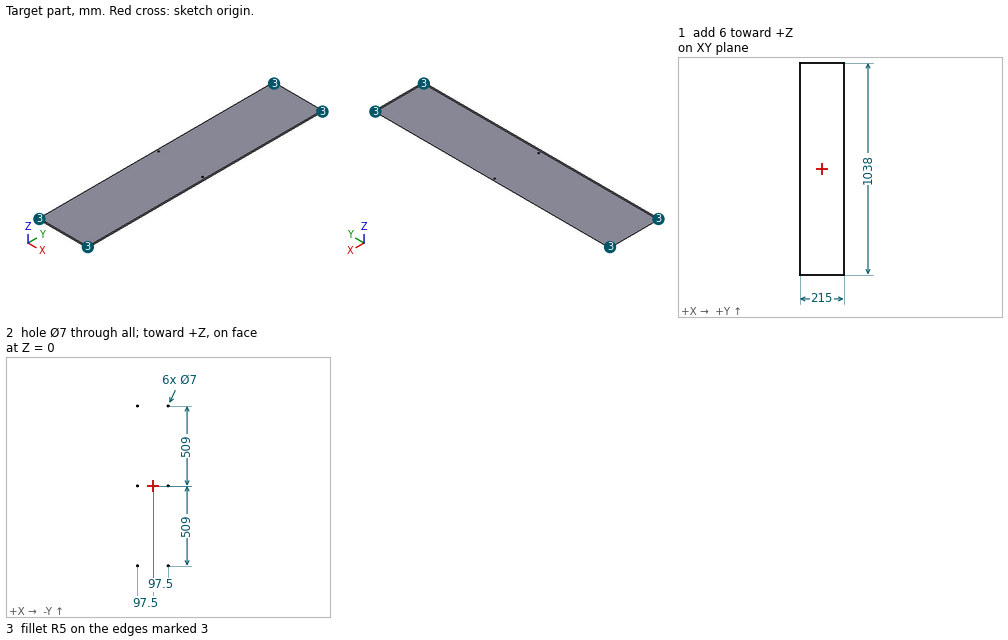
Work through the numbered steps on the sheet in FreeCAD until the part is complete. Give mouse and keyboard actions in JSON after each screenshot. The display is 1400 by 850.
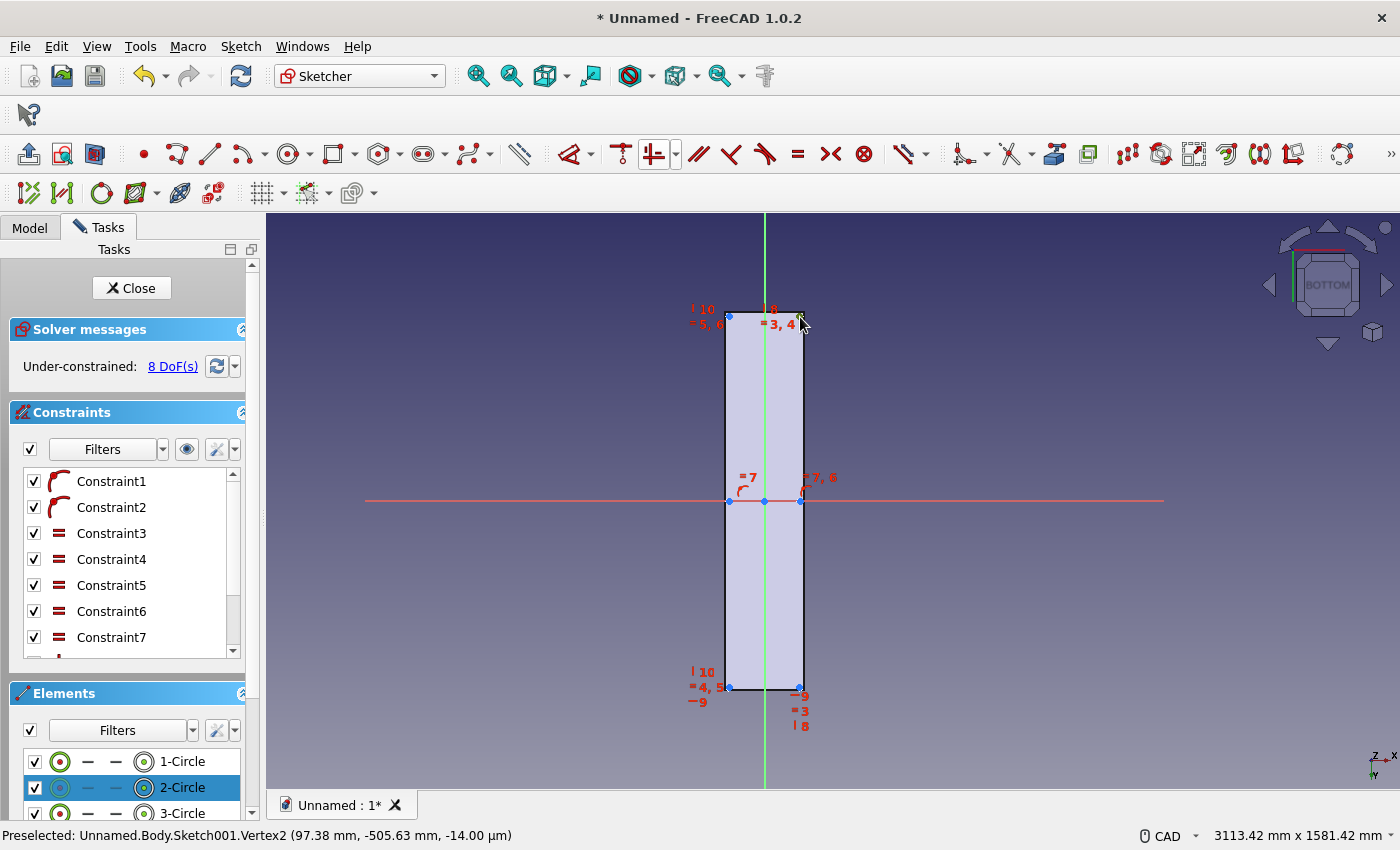
{"action": "left_click", "coordinate": [729, 317]}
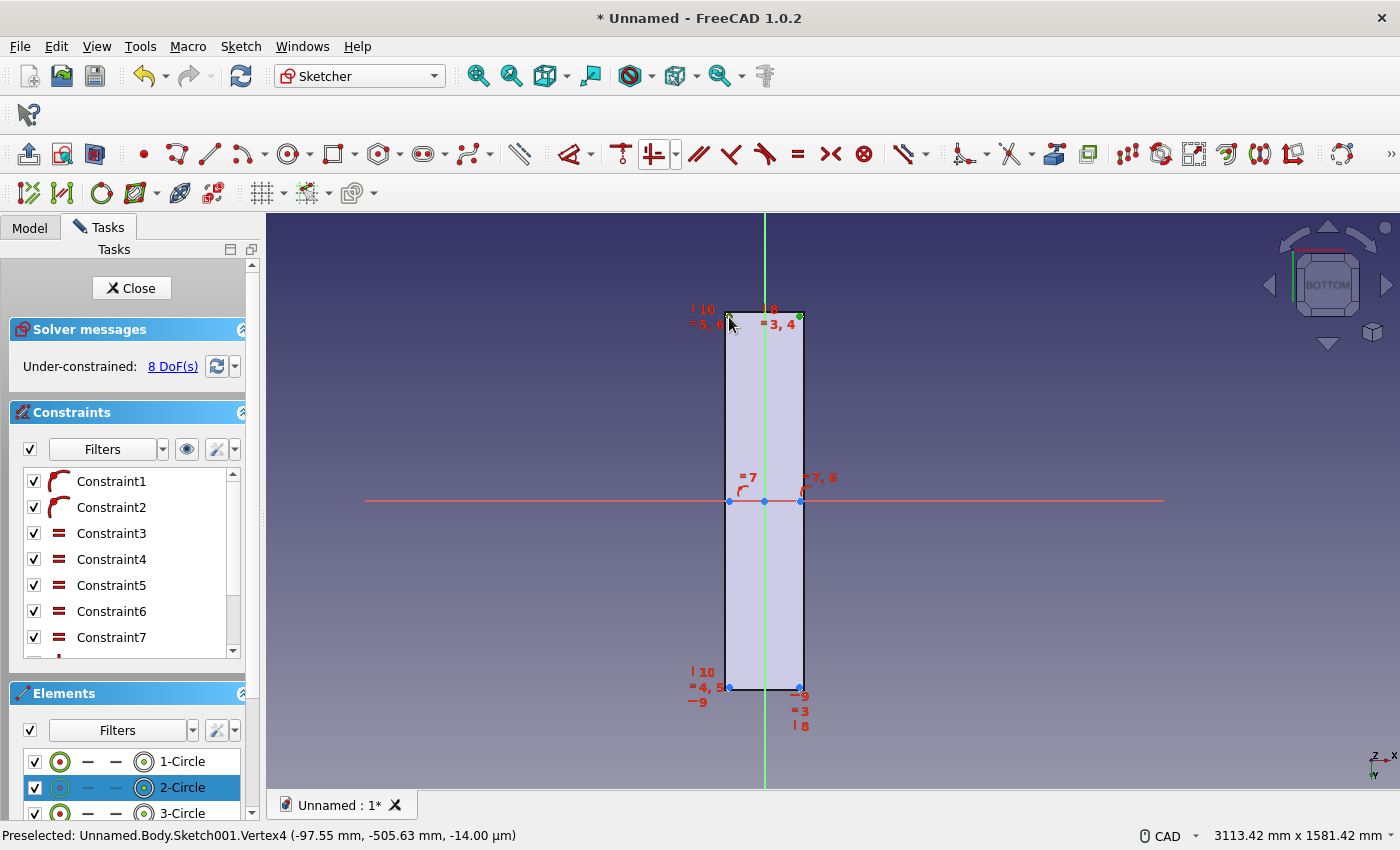
{"action": "left_click", "coordinate": [676, 154]}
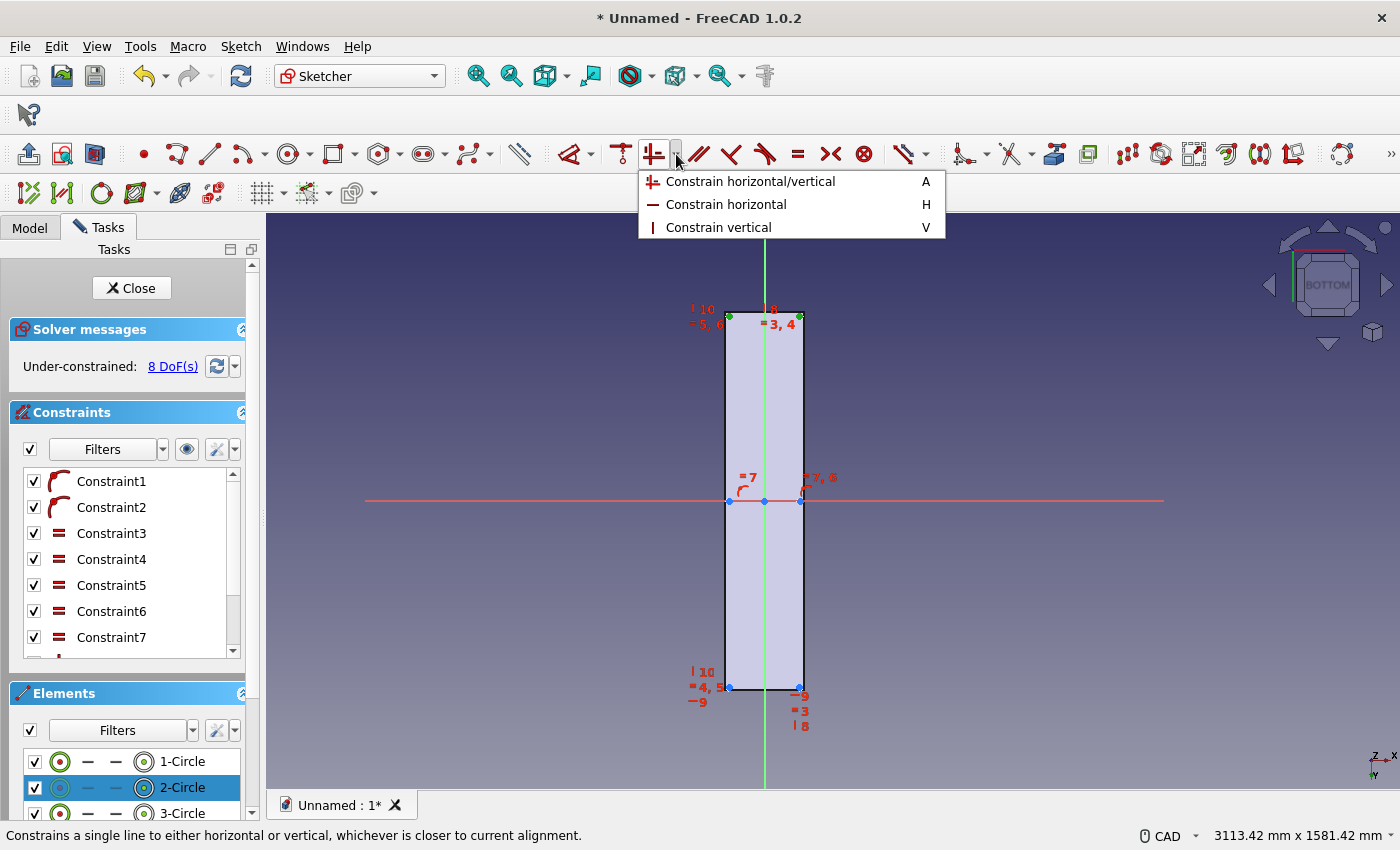
{"action": "left_click", "coordinate": [792, 204]}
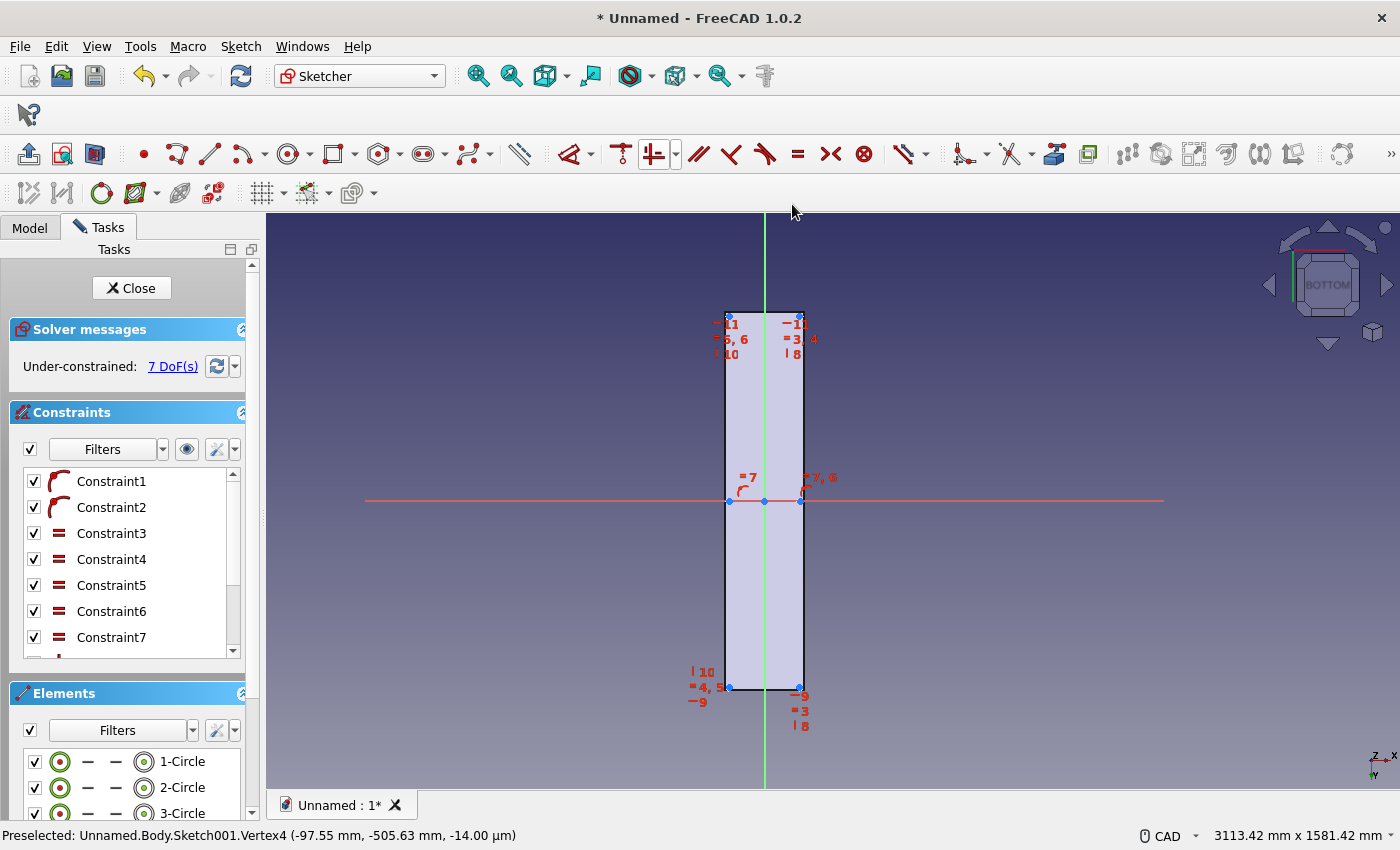
{"action": "left_click", "coordinate": [800, 688]}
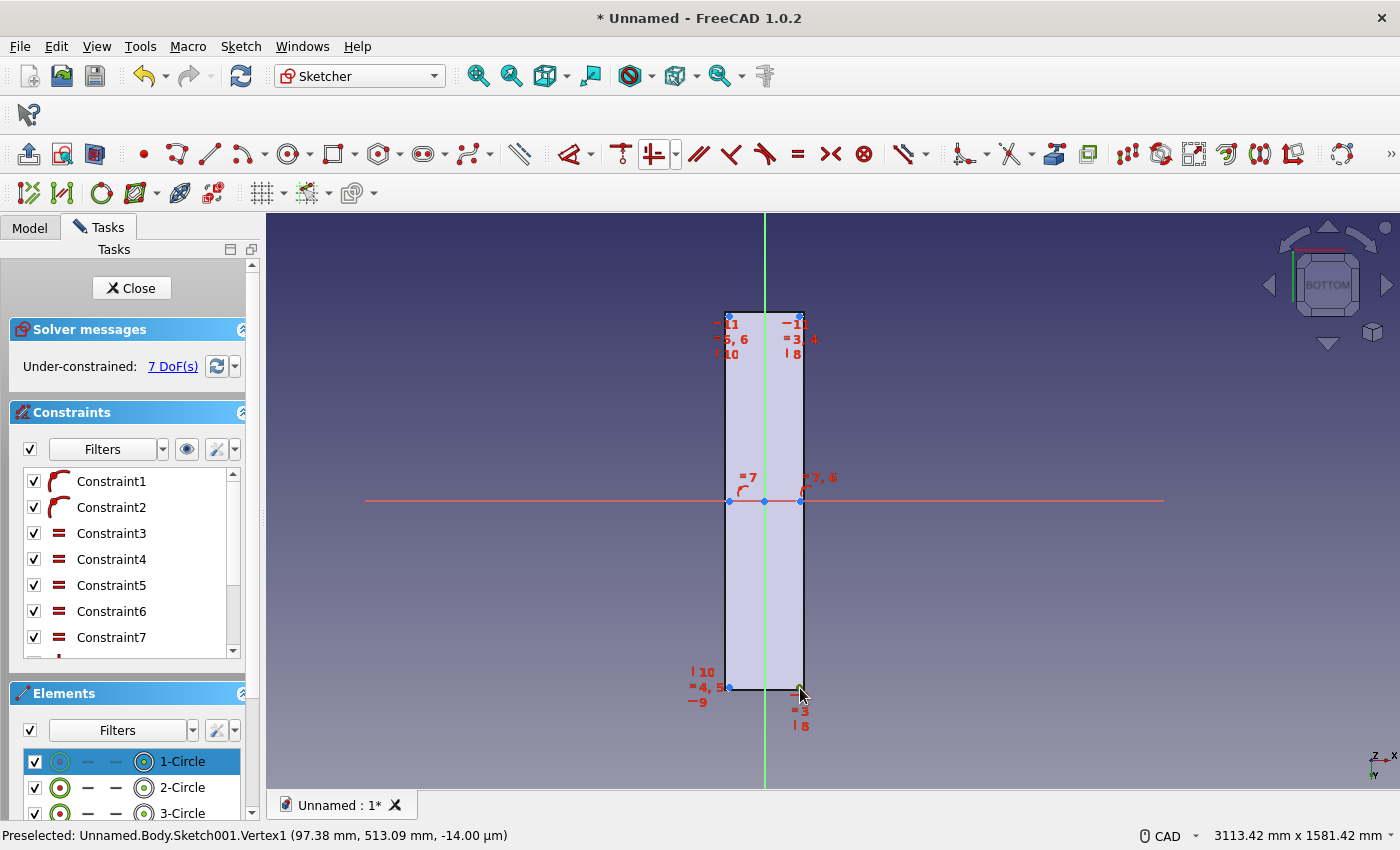
{"action": "left_click", "coordinate": [800, 501]}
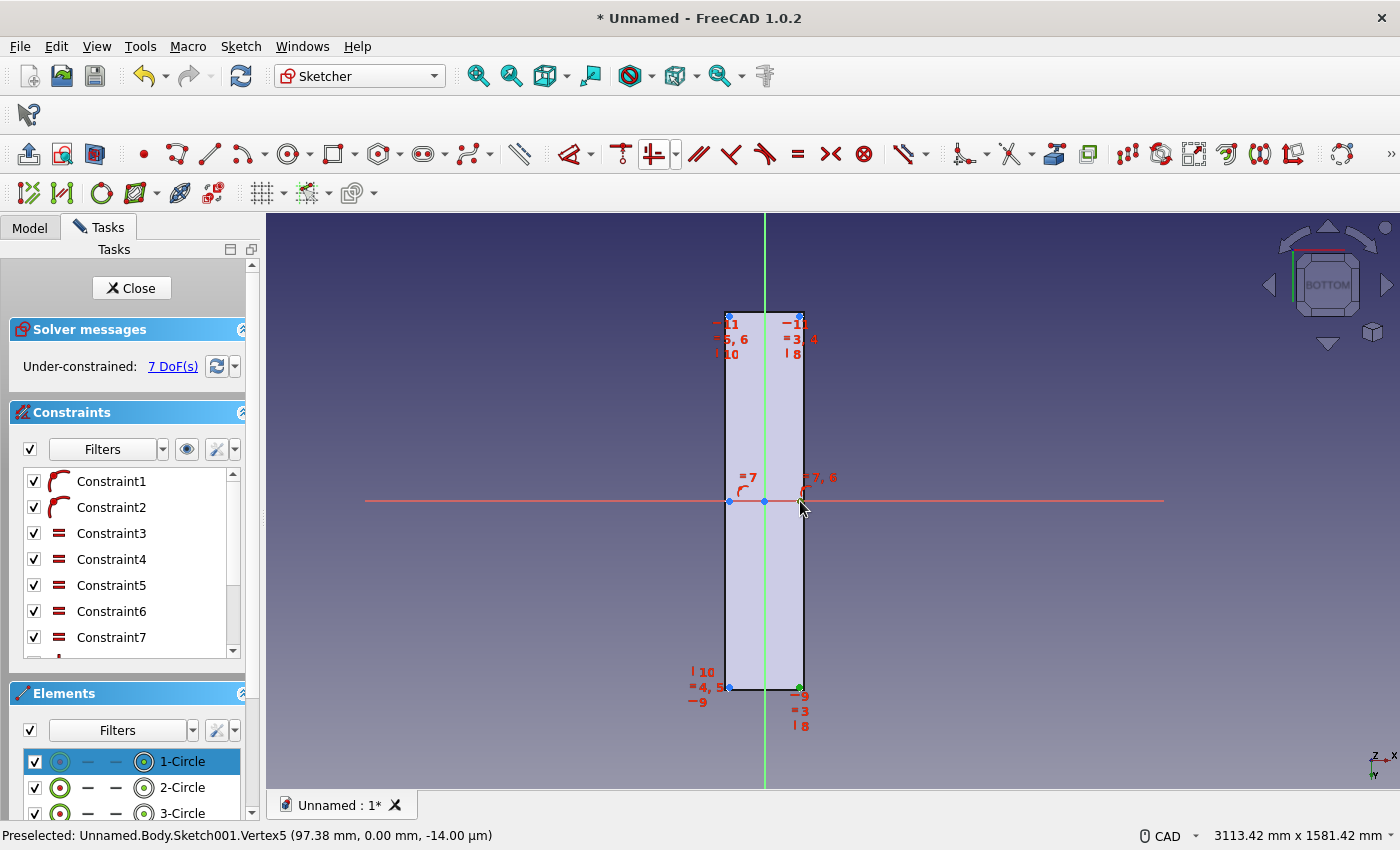
{"action": "key", "text": "v"}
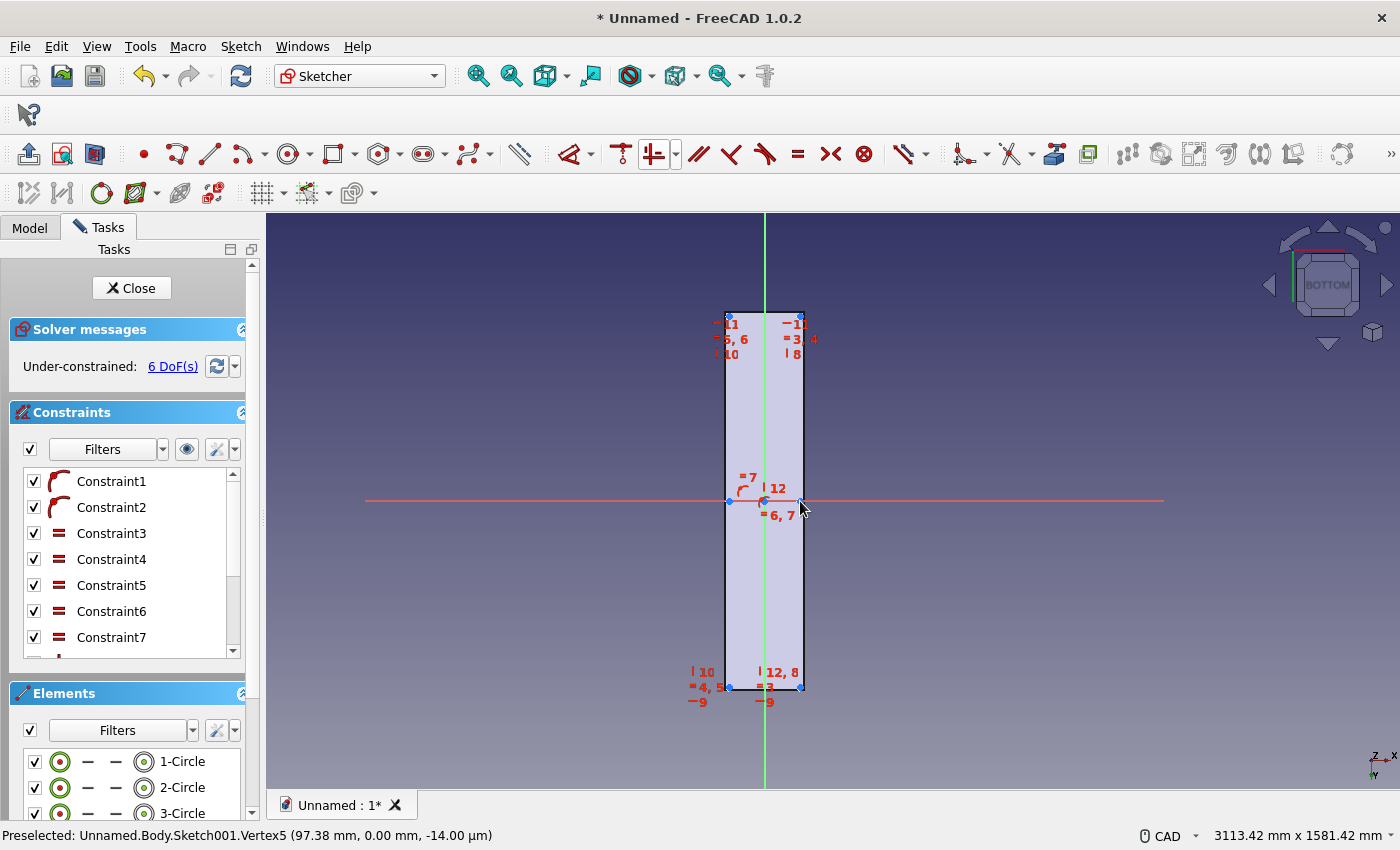
{"action": "left_click", "coordinate": [729, 688]}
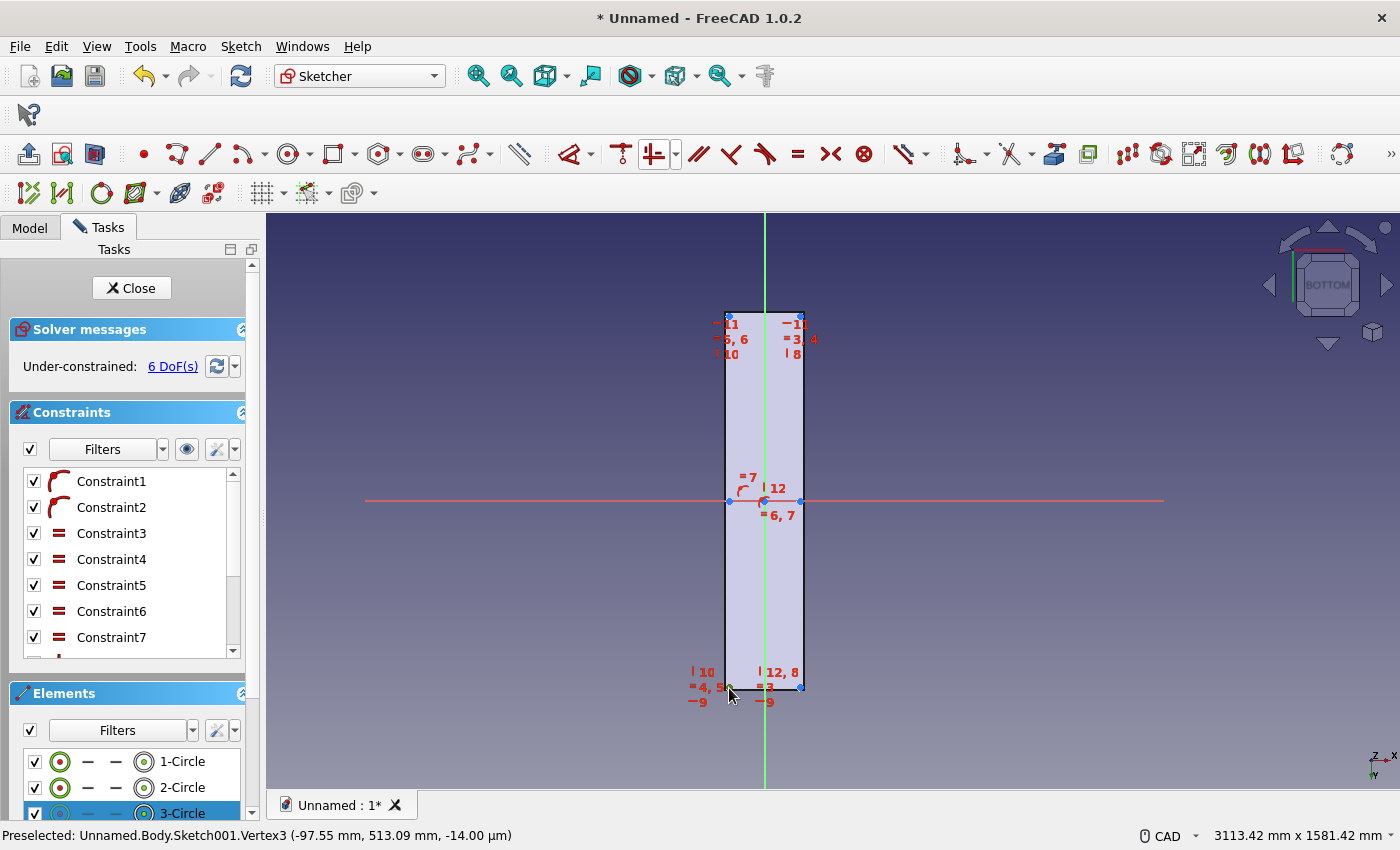
{"action": "left_click", "coordinate": [729, 501]}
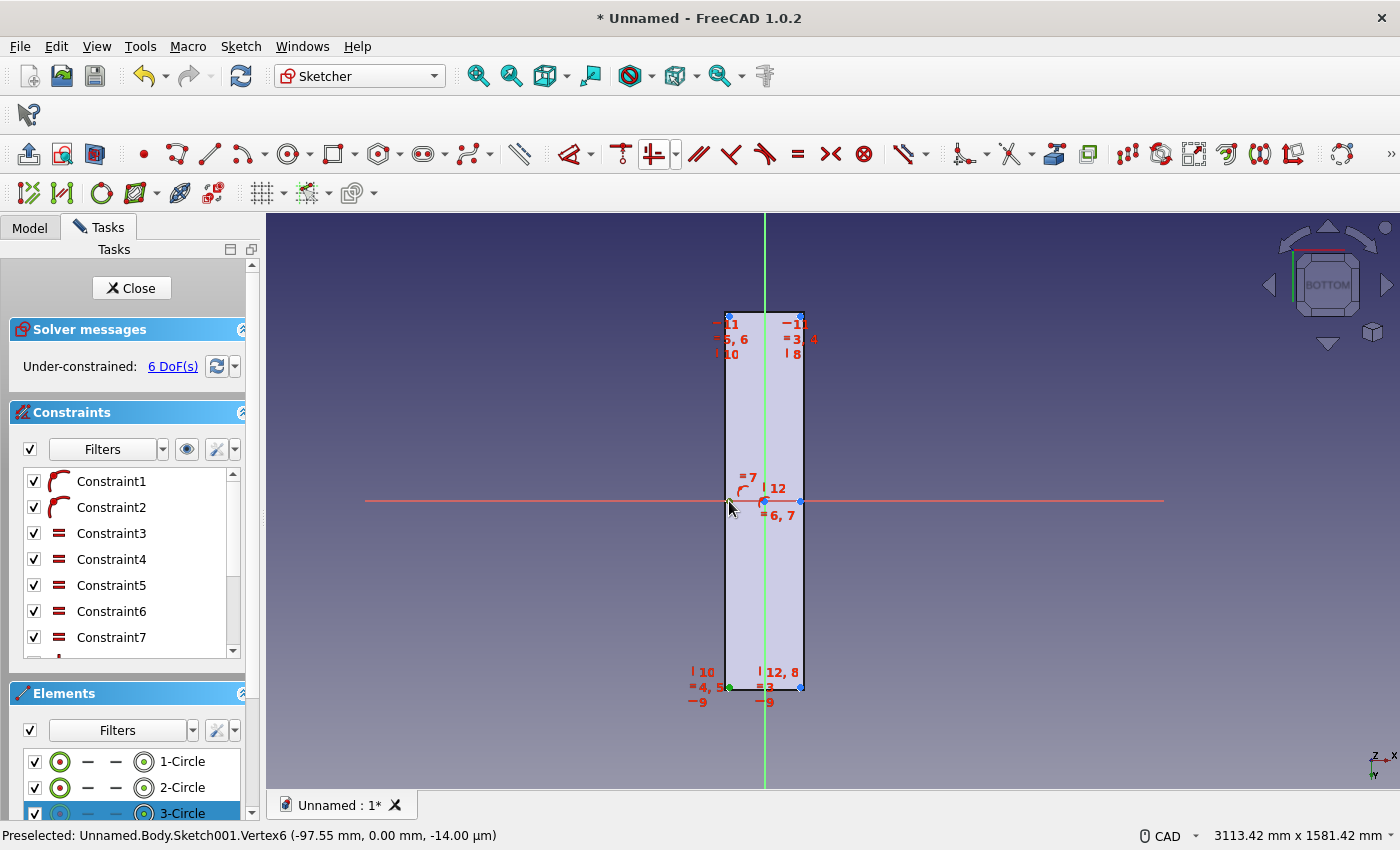
{"action": "key", "text": "v"}